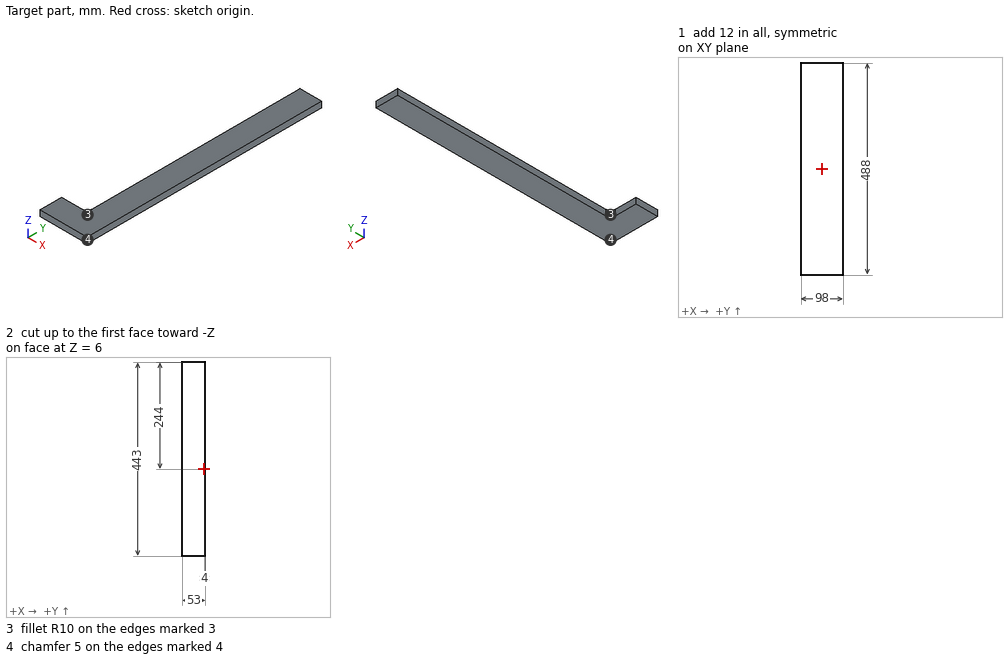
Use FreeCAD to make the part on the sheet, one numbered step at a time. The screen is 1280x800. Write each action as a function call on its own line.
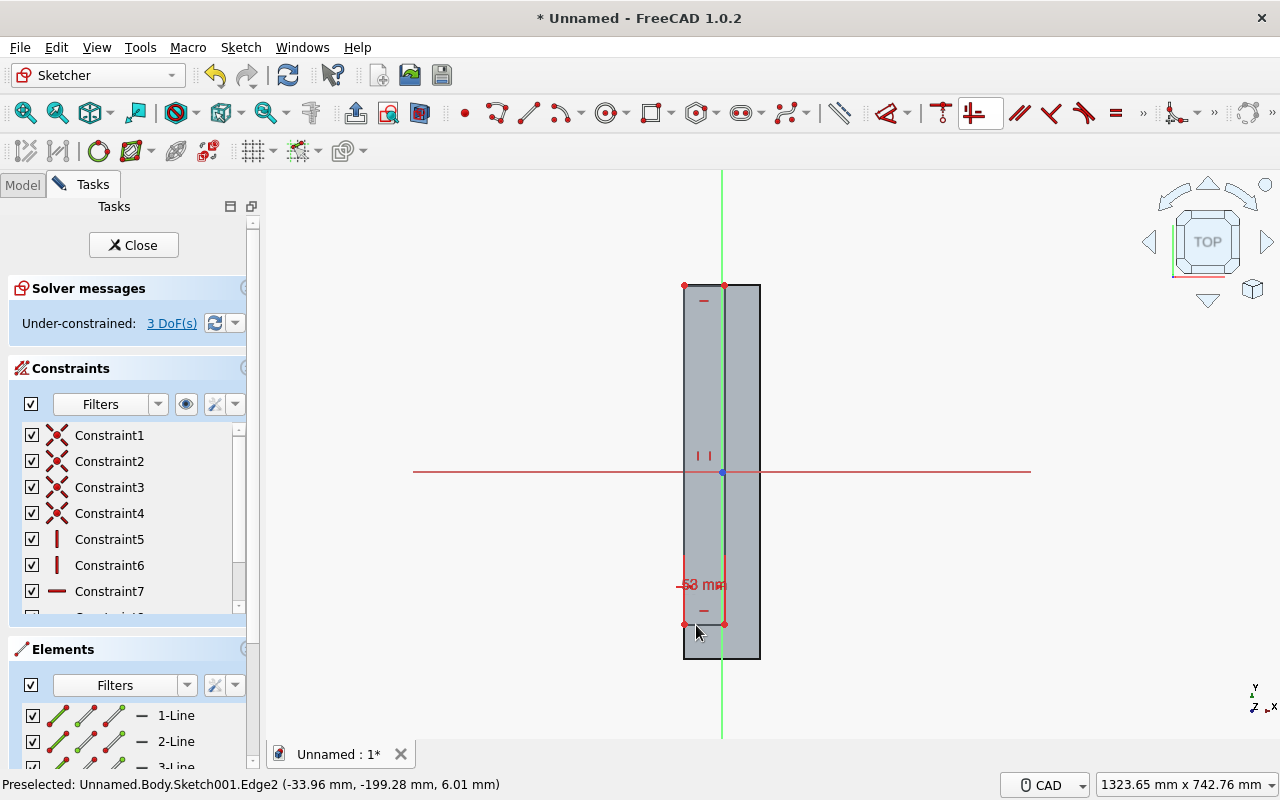
scroll(725, 625, up, 13)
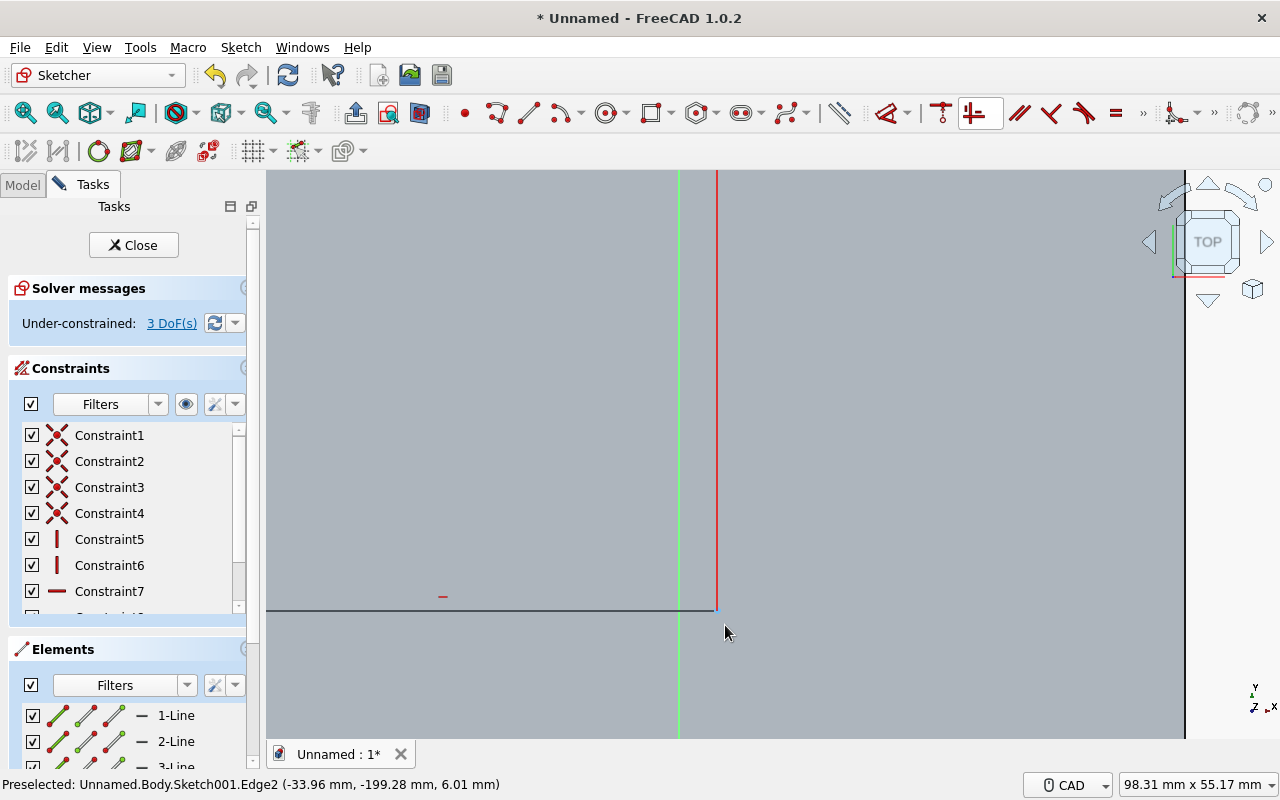
click(717, 611)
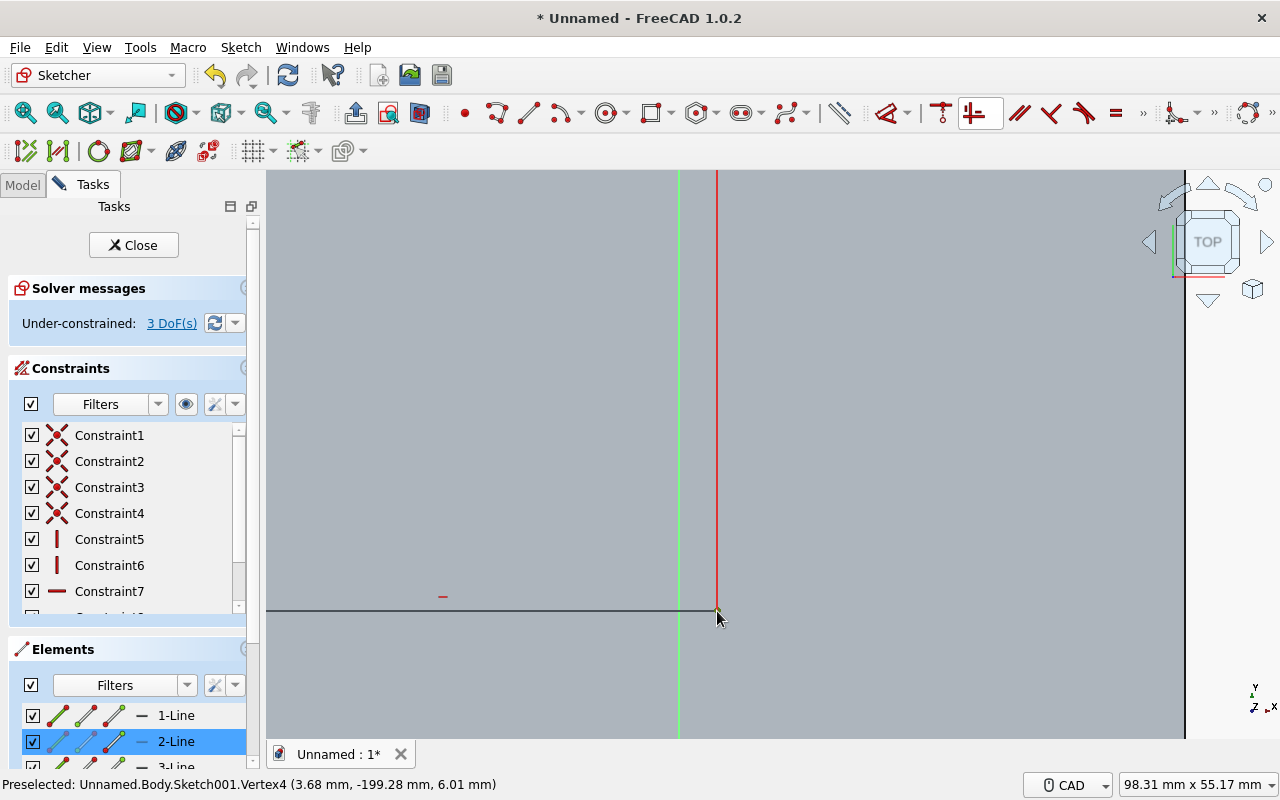
key(l)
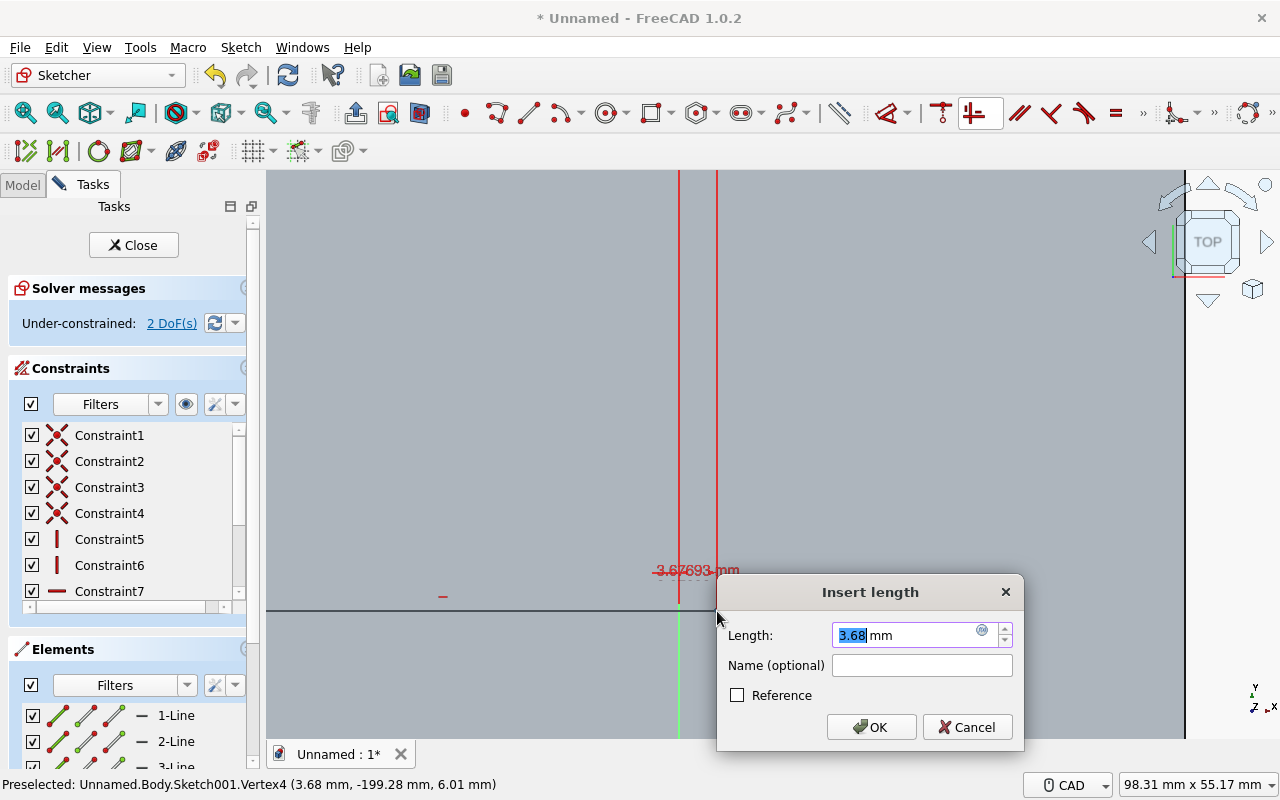
text(4)
key(Return)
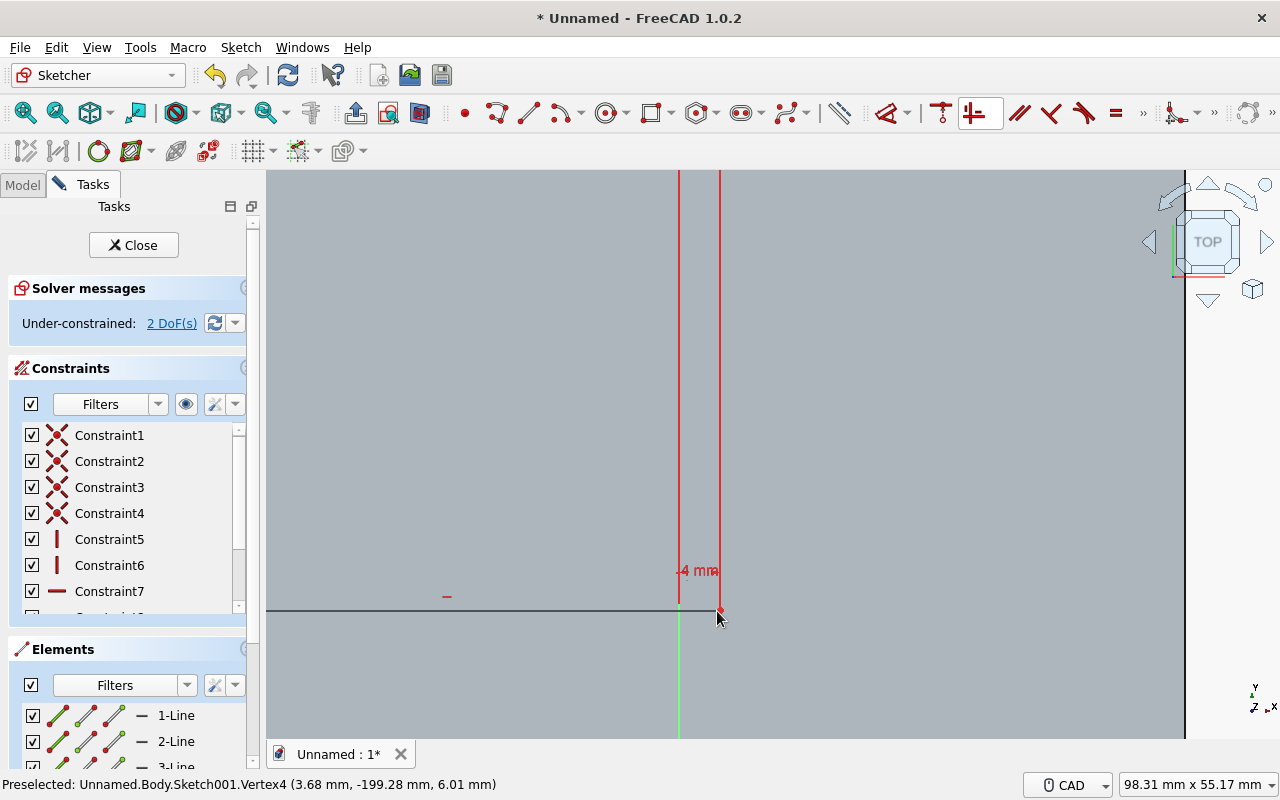
scroll(725, 626, down, 13)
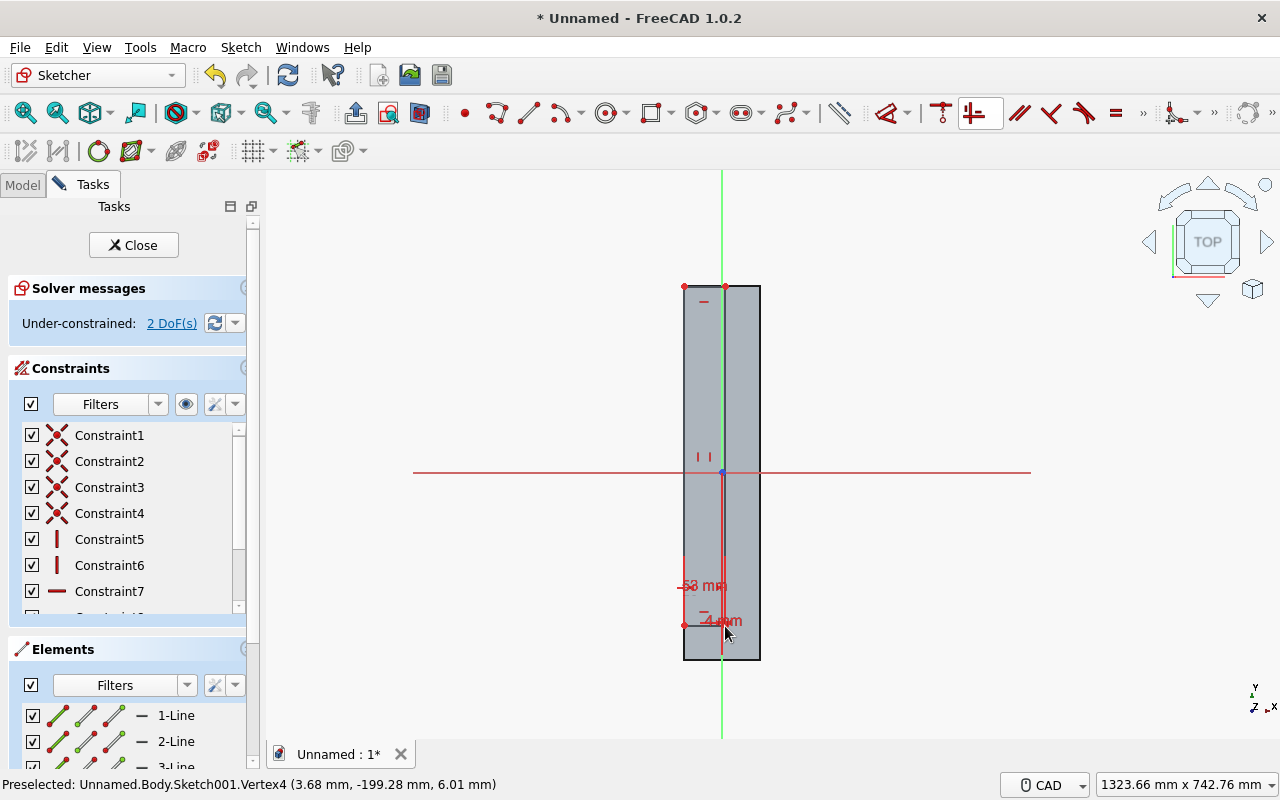
click(684, 389)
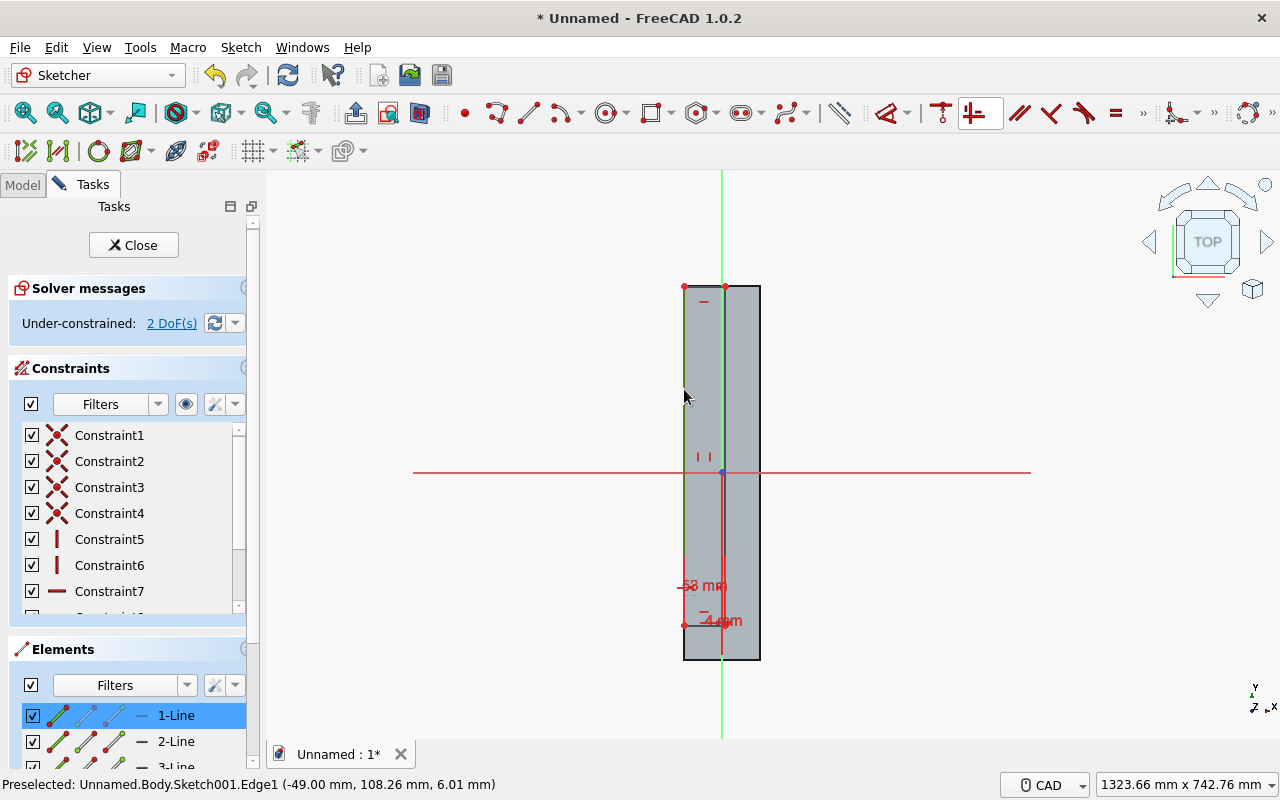
key(i)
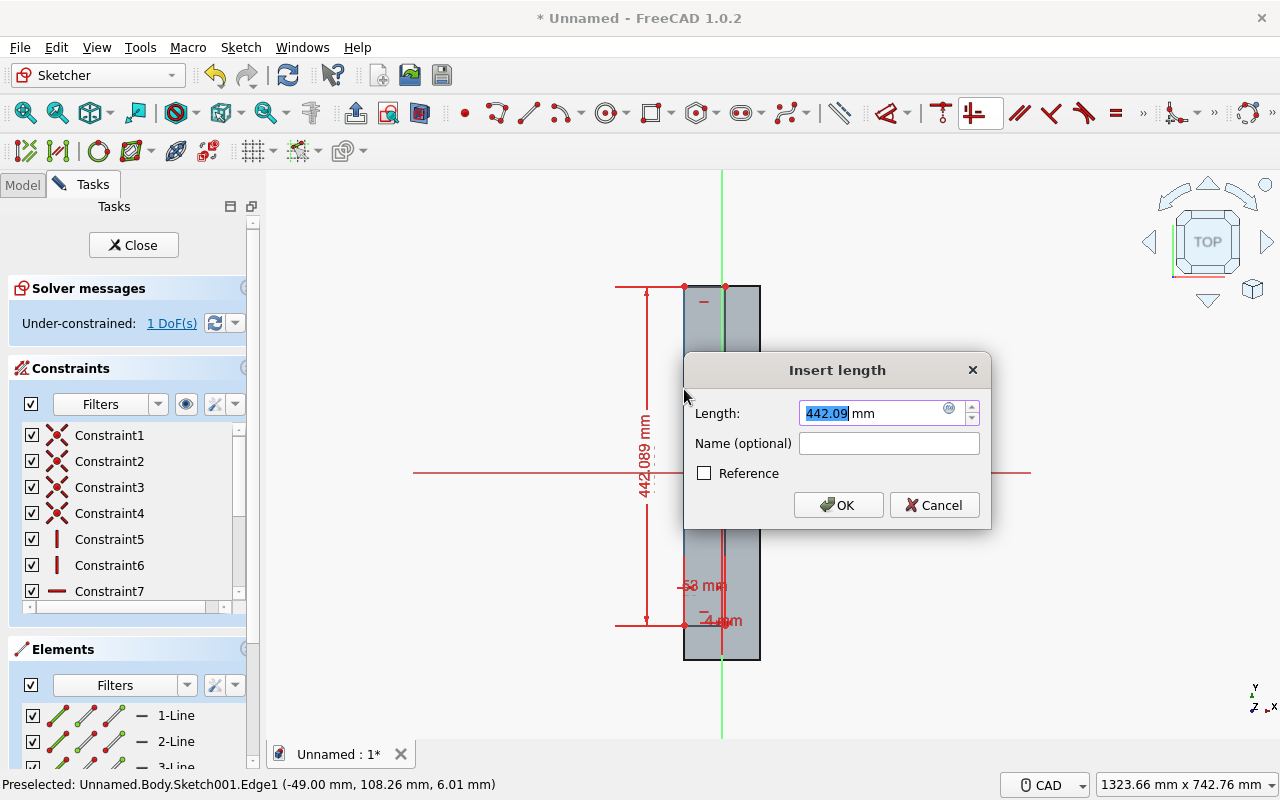
text(443)
key(Return)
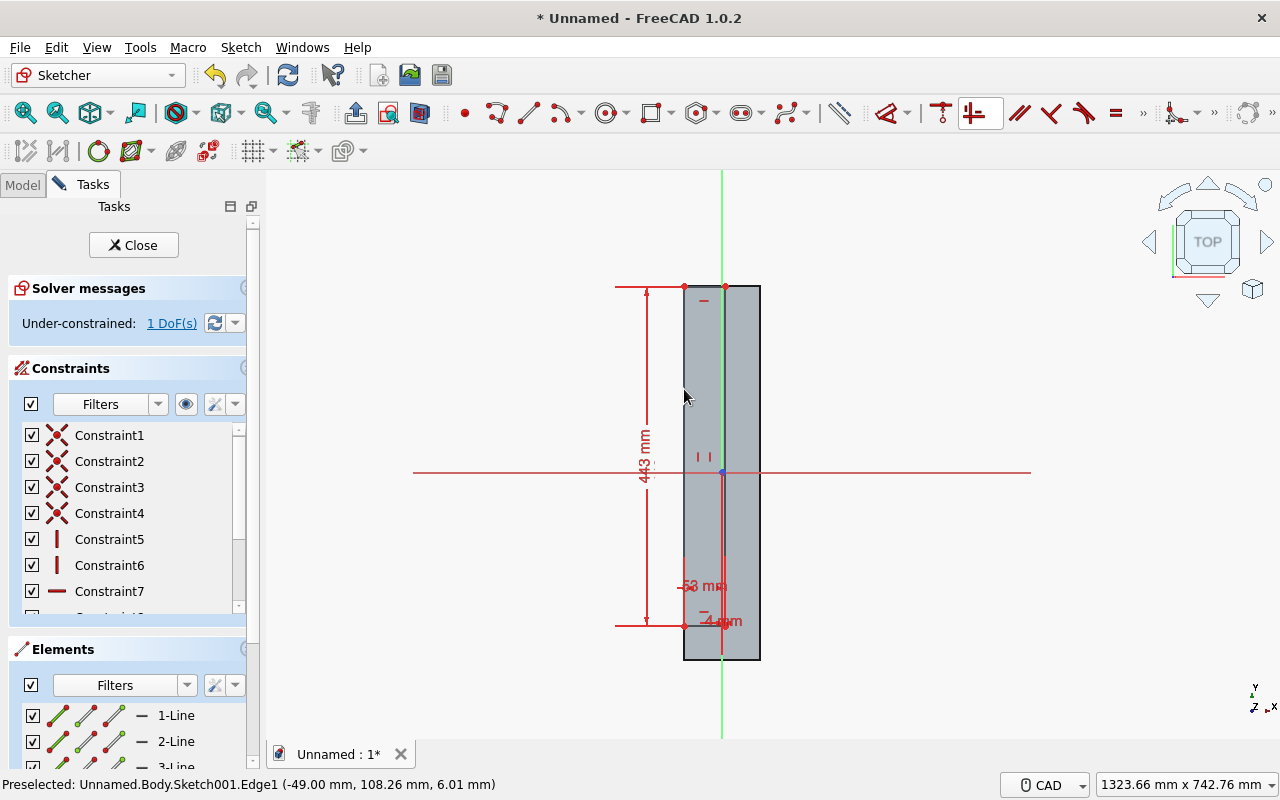
click(684, 287)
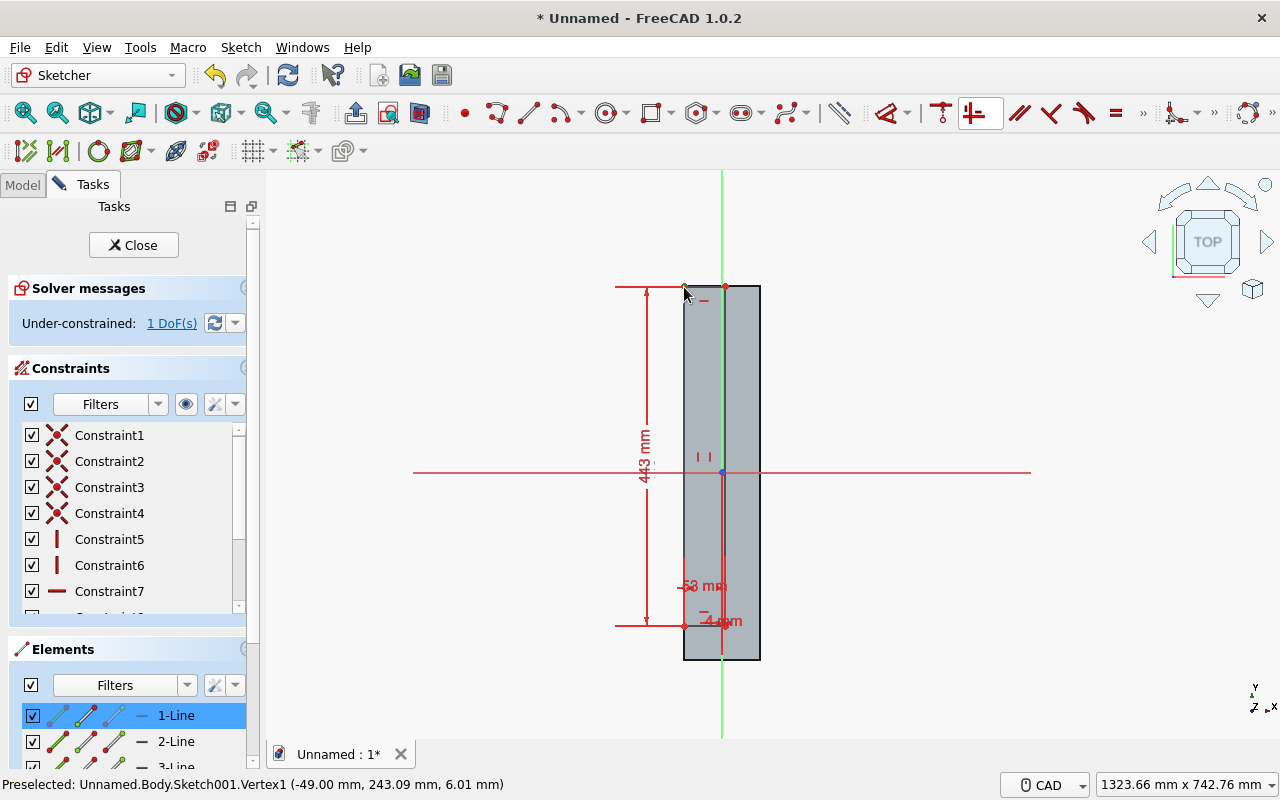
key(i)